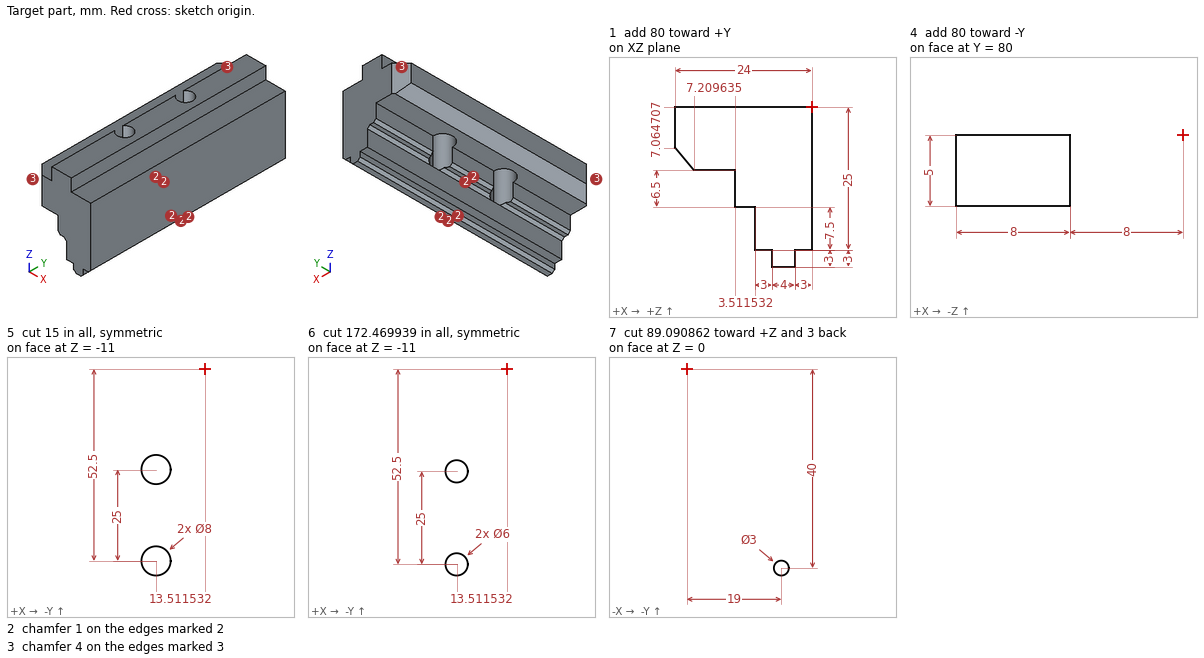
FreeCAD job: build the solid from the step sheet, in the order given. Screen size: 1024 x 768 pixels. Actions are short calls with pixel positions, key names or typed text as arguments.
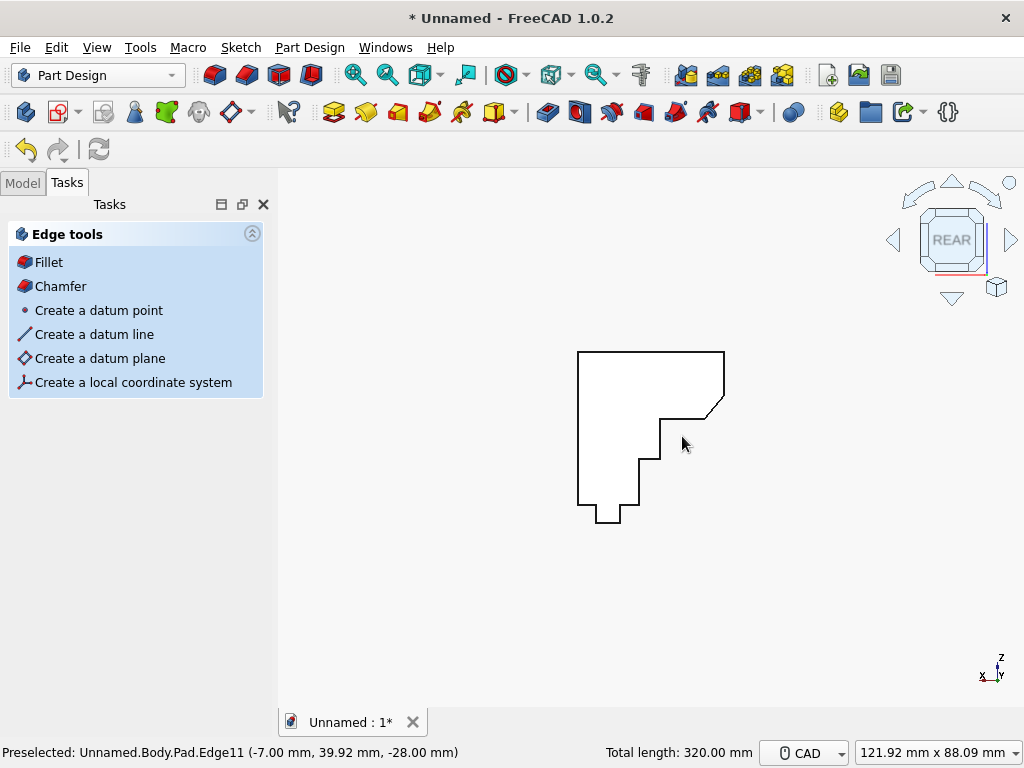
key(v)
key(f)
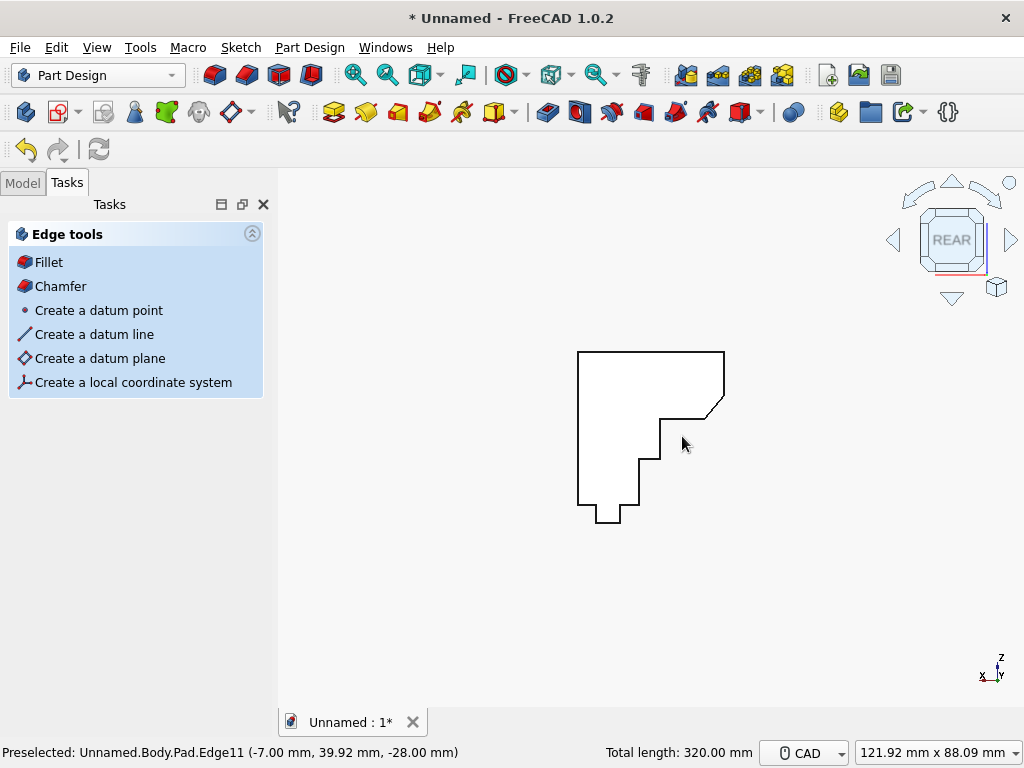
key(6)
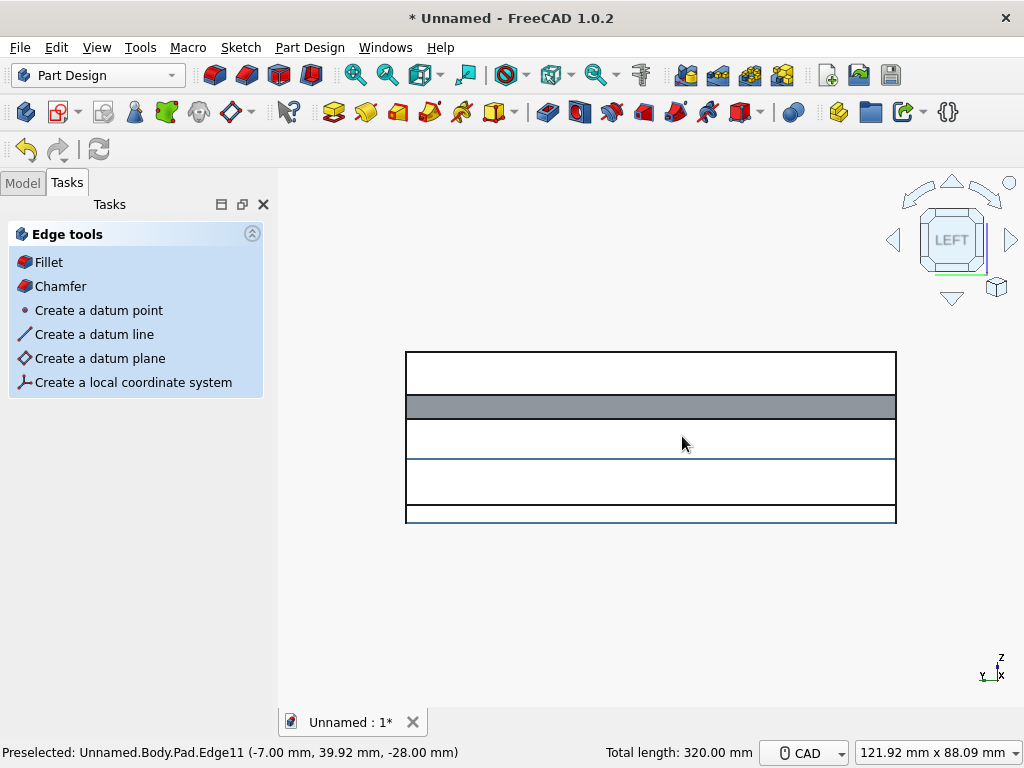
key(v)
key(3)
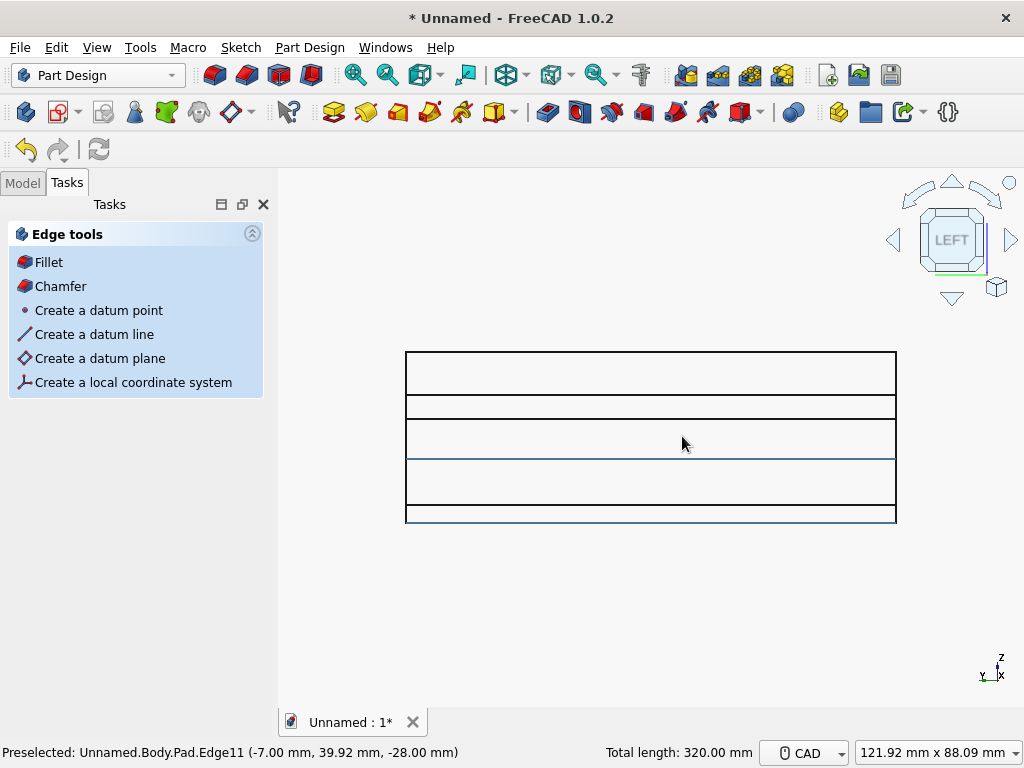
key(0)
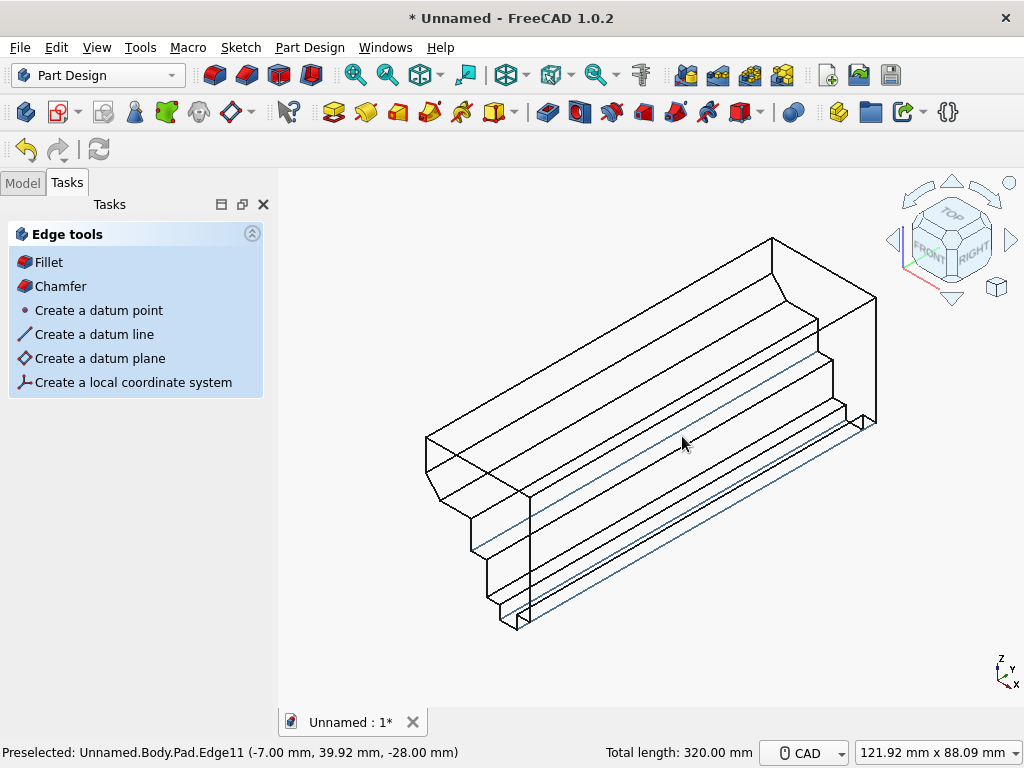
click(660, 459, ctrl)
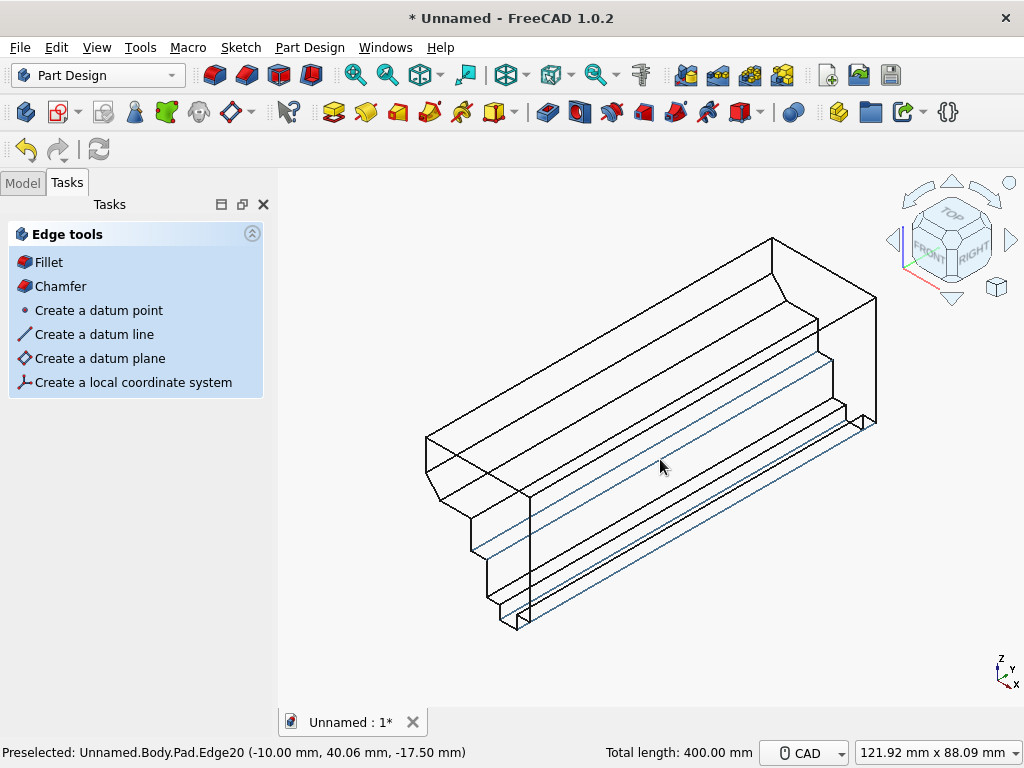
key(v)
key(1)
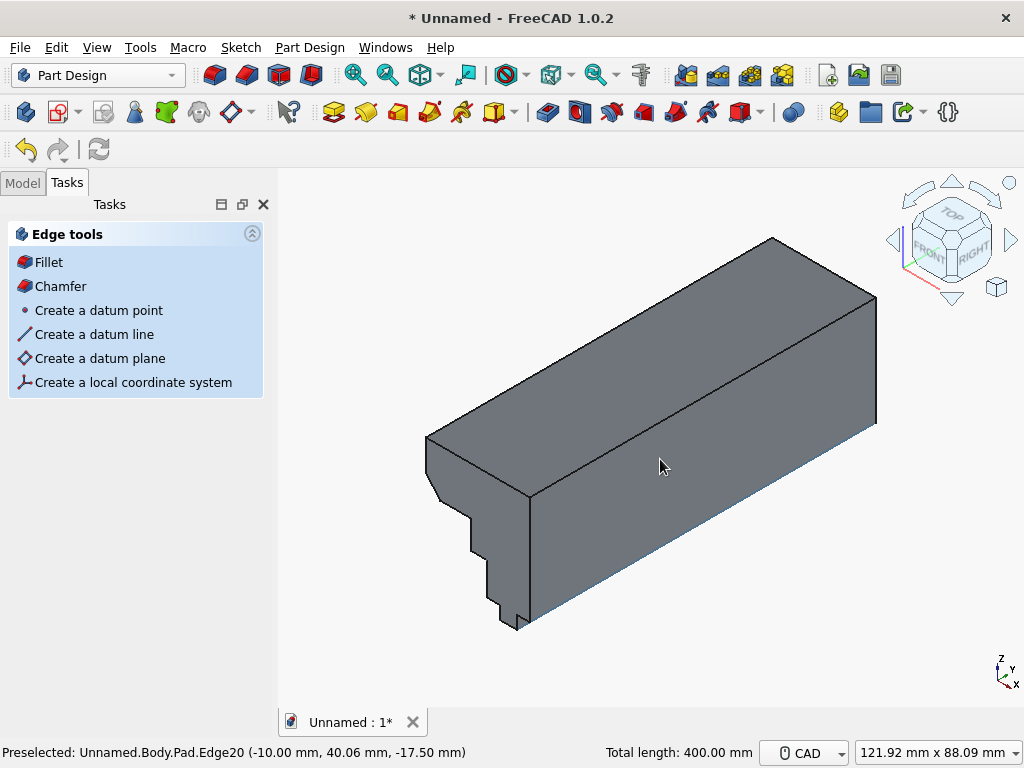
click(248, 76)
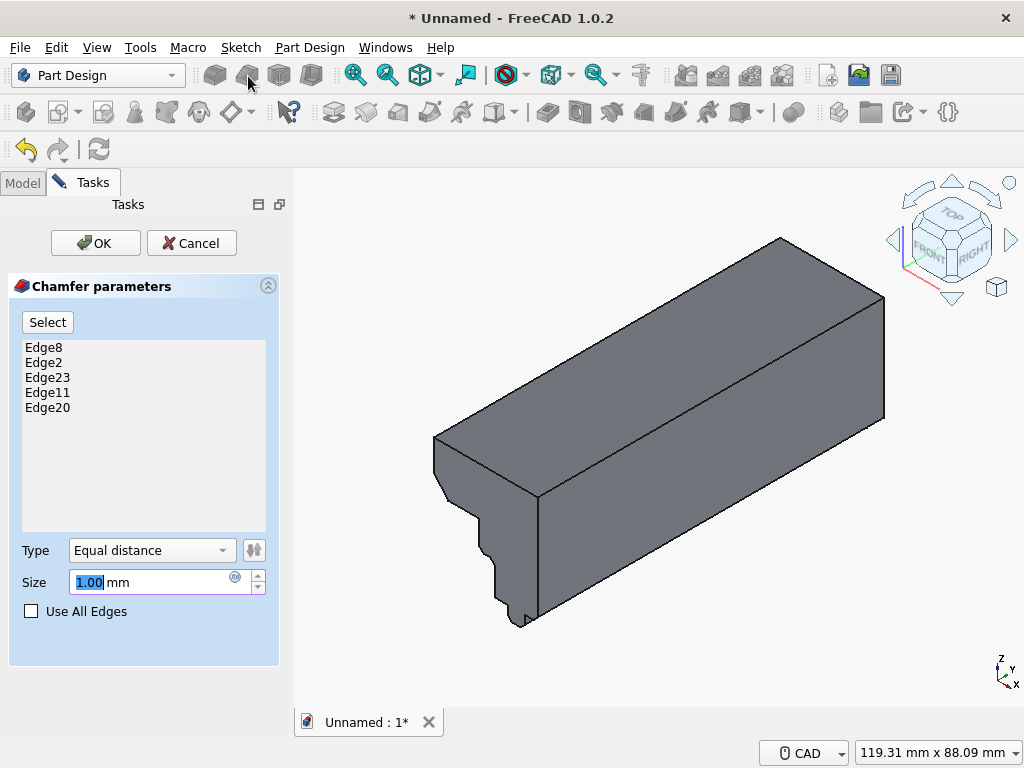
text(1)
key(Tab)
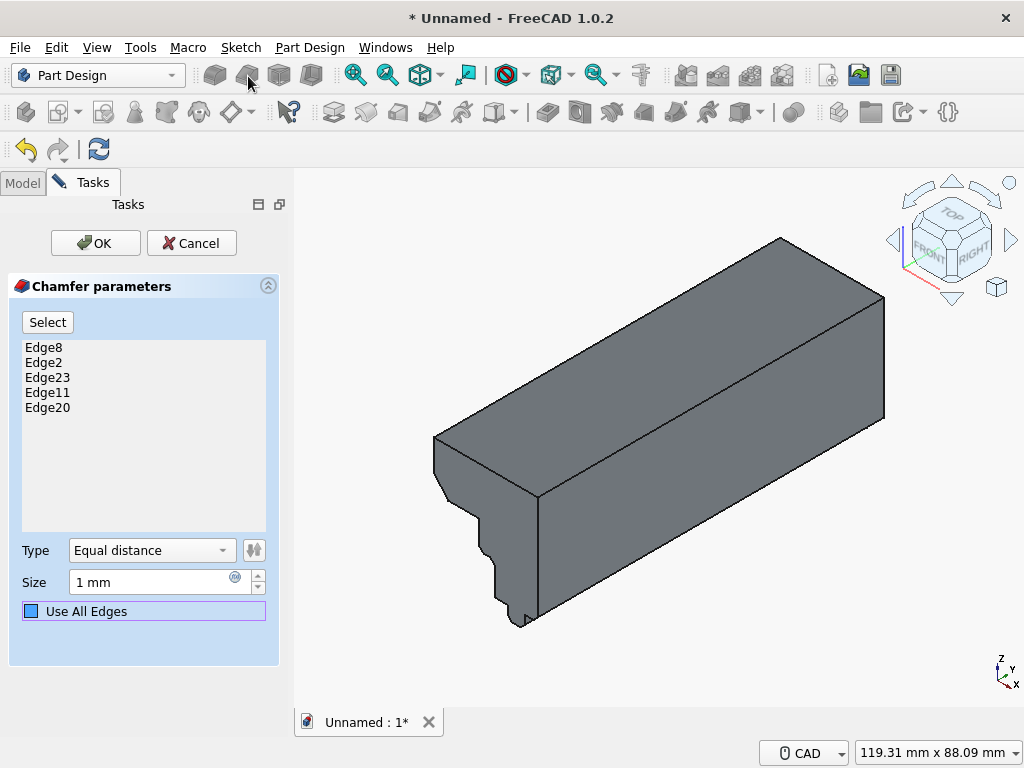
click(96, 243)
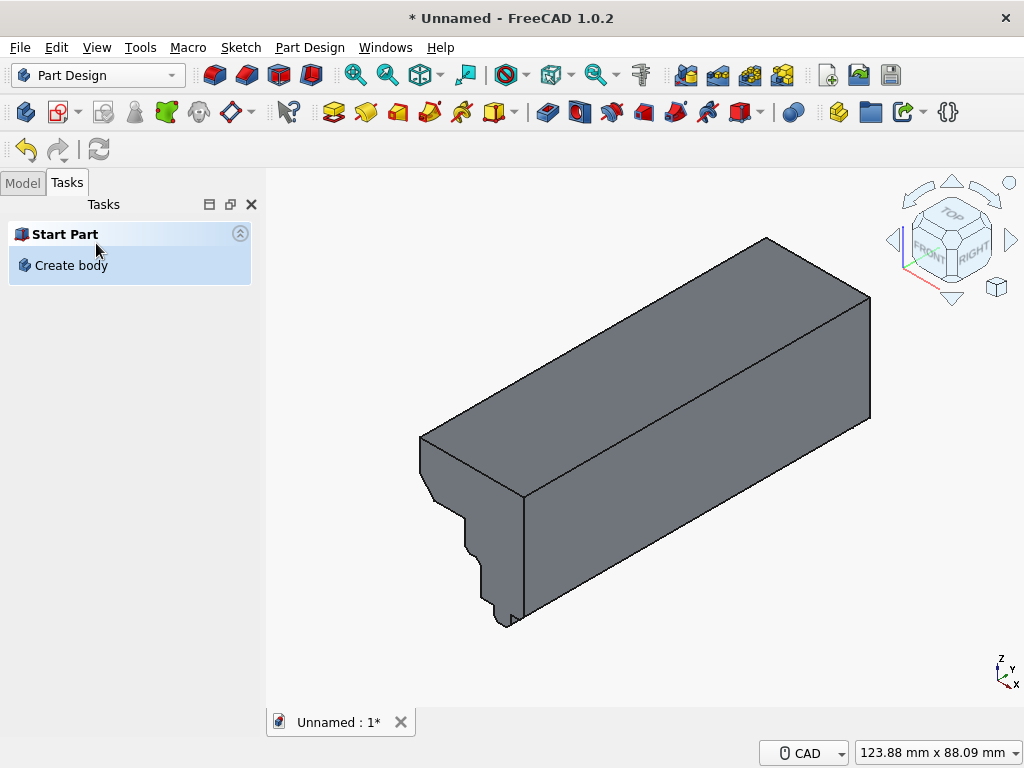
key(2)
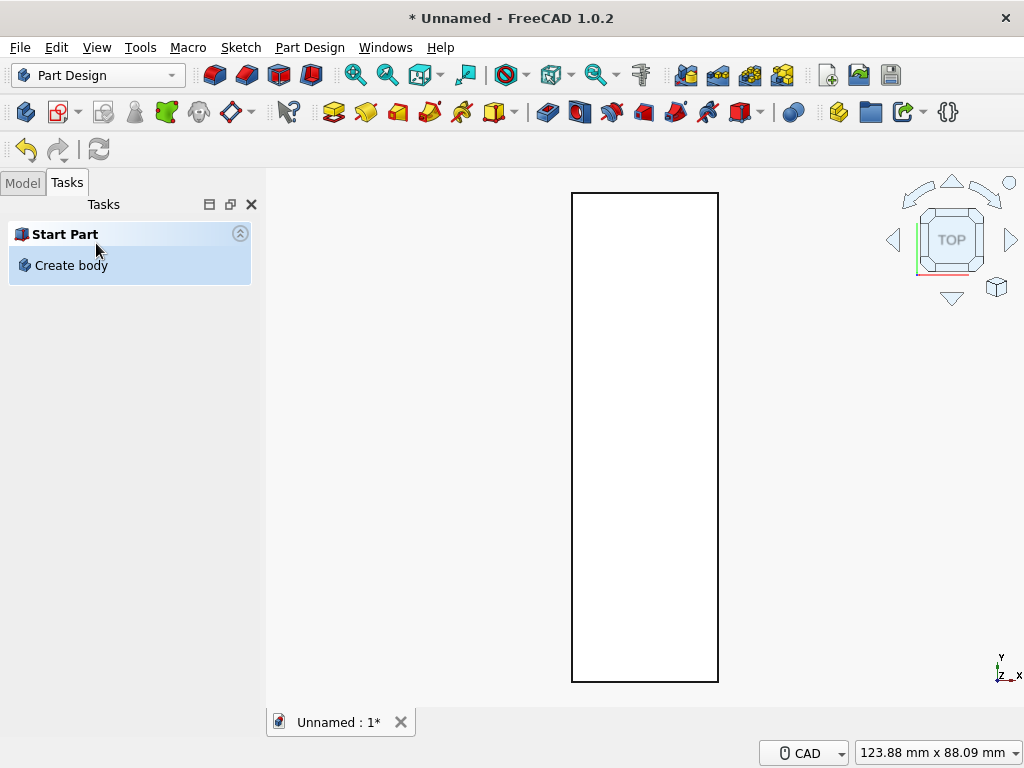
key(0)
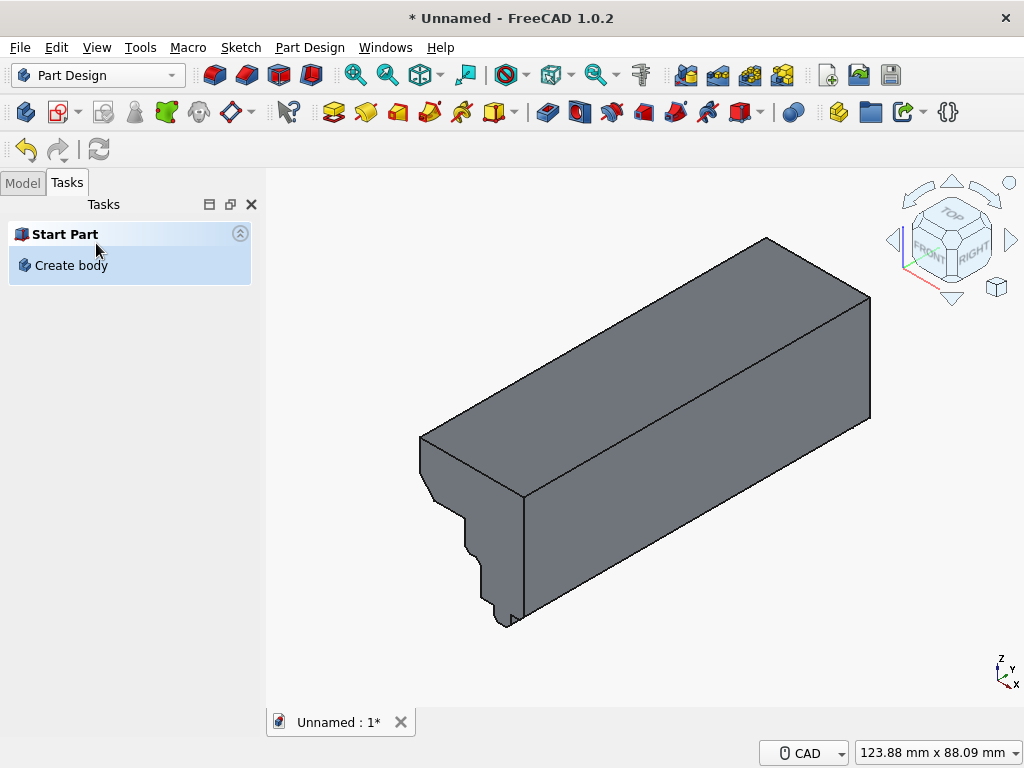
key(1)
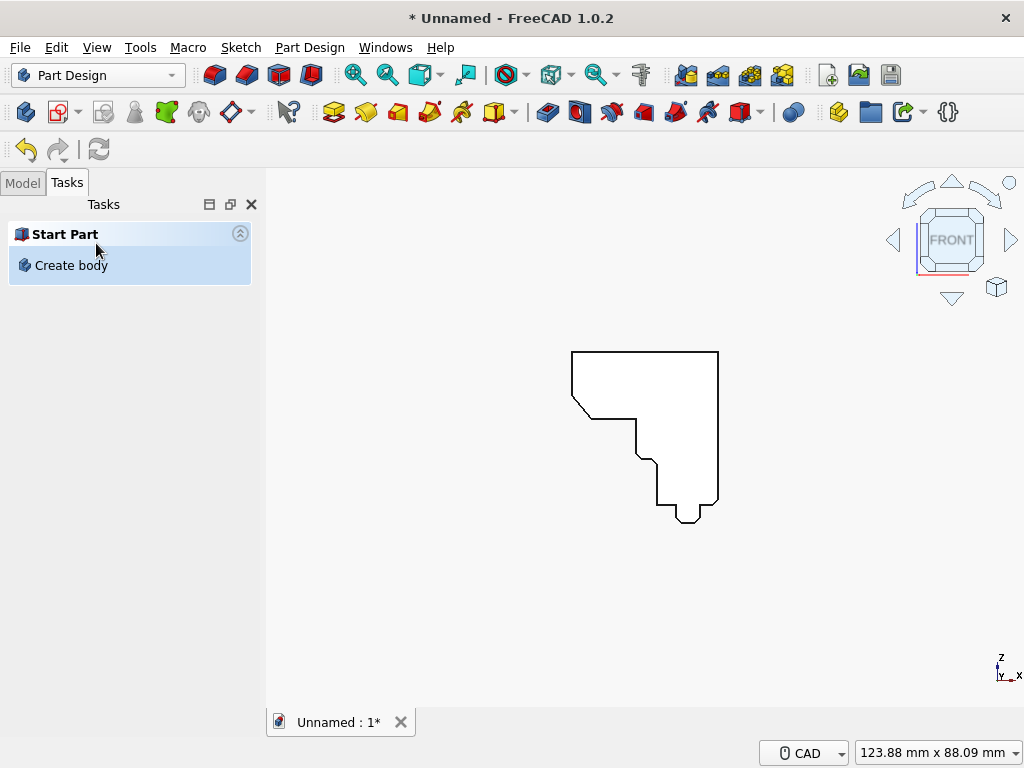
key(v)
key(f)